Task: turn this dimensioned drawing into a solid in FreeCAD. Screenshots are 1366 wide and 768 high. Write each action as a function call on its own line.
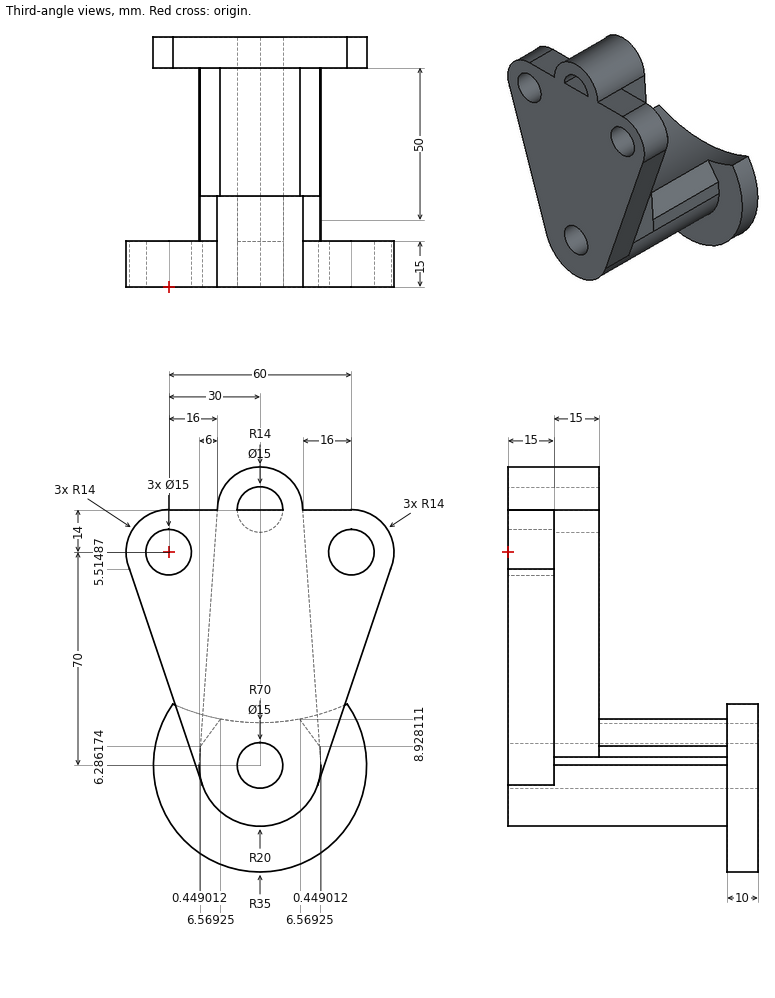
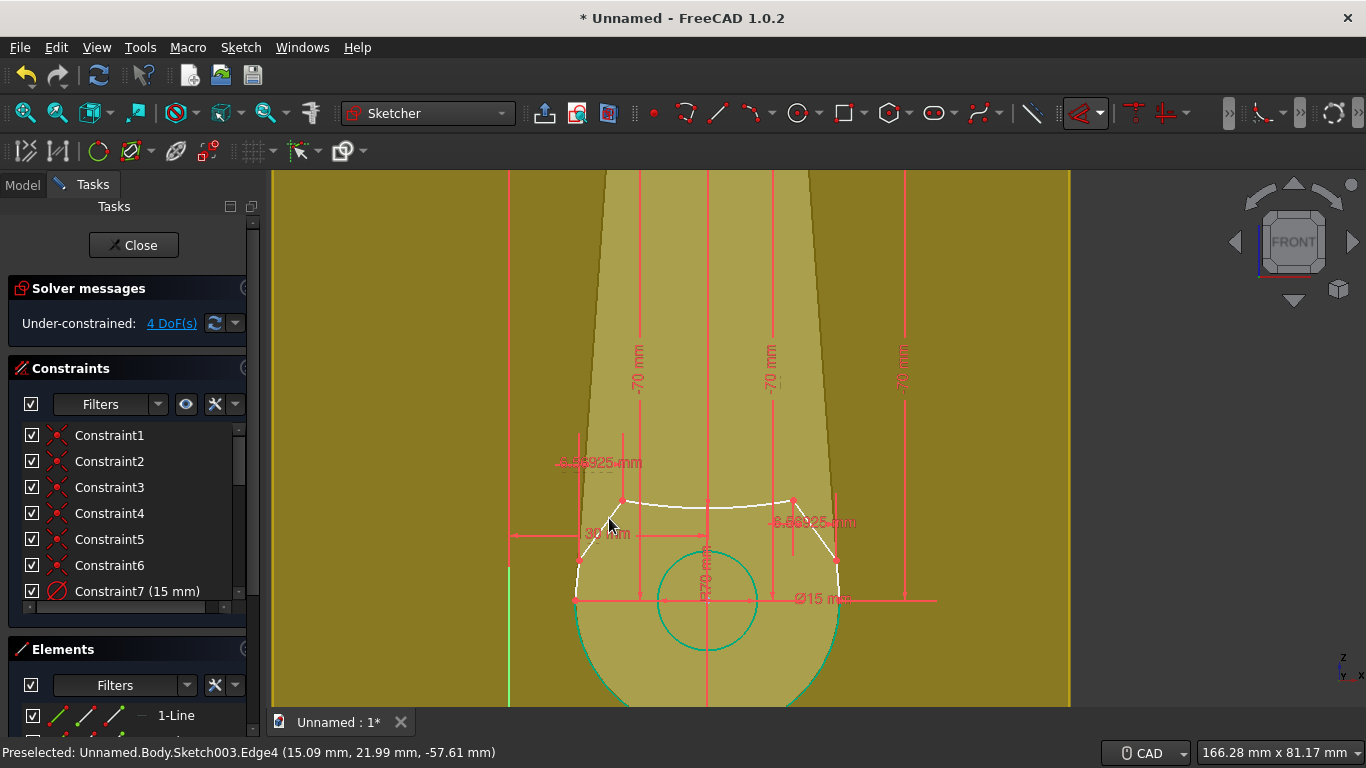
click(823, 542)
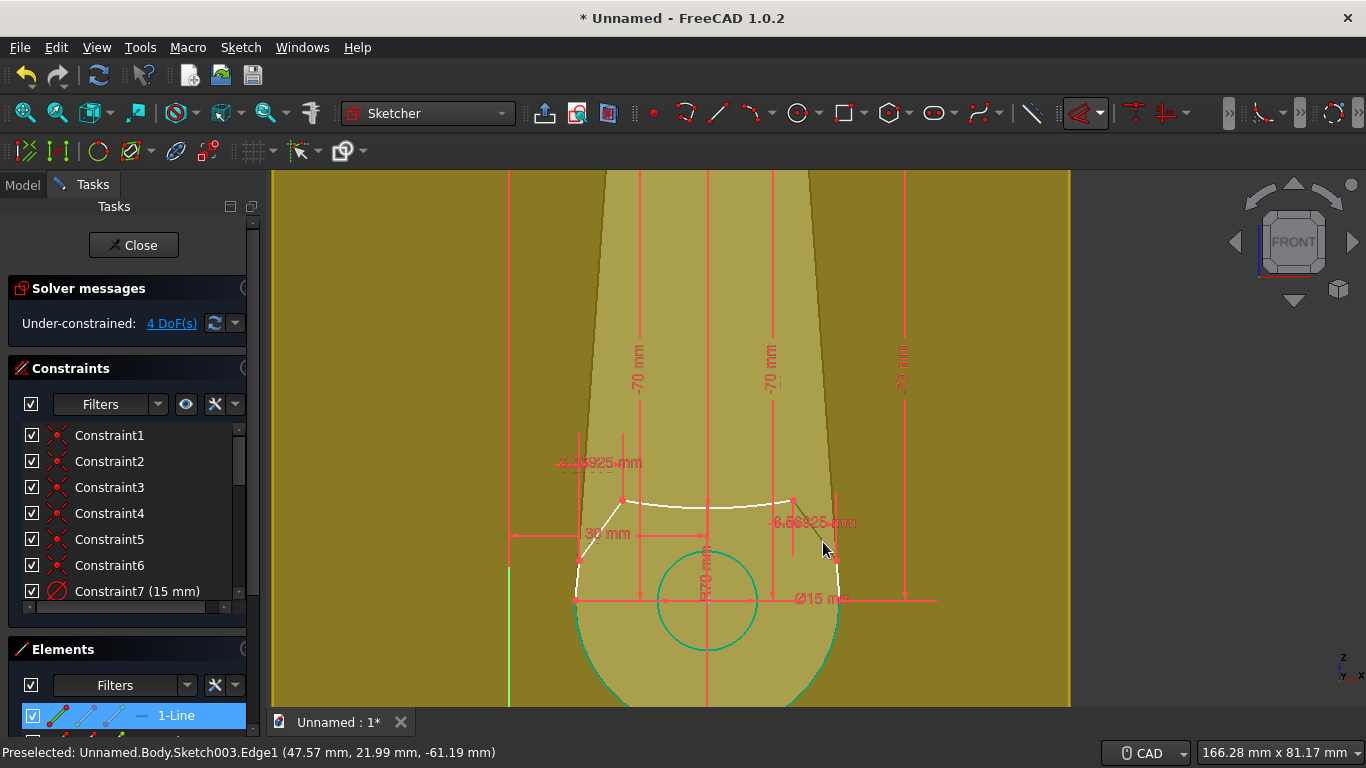
click(1102, 114)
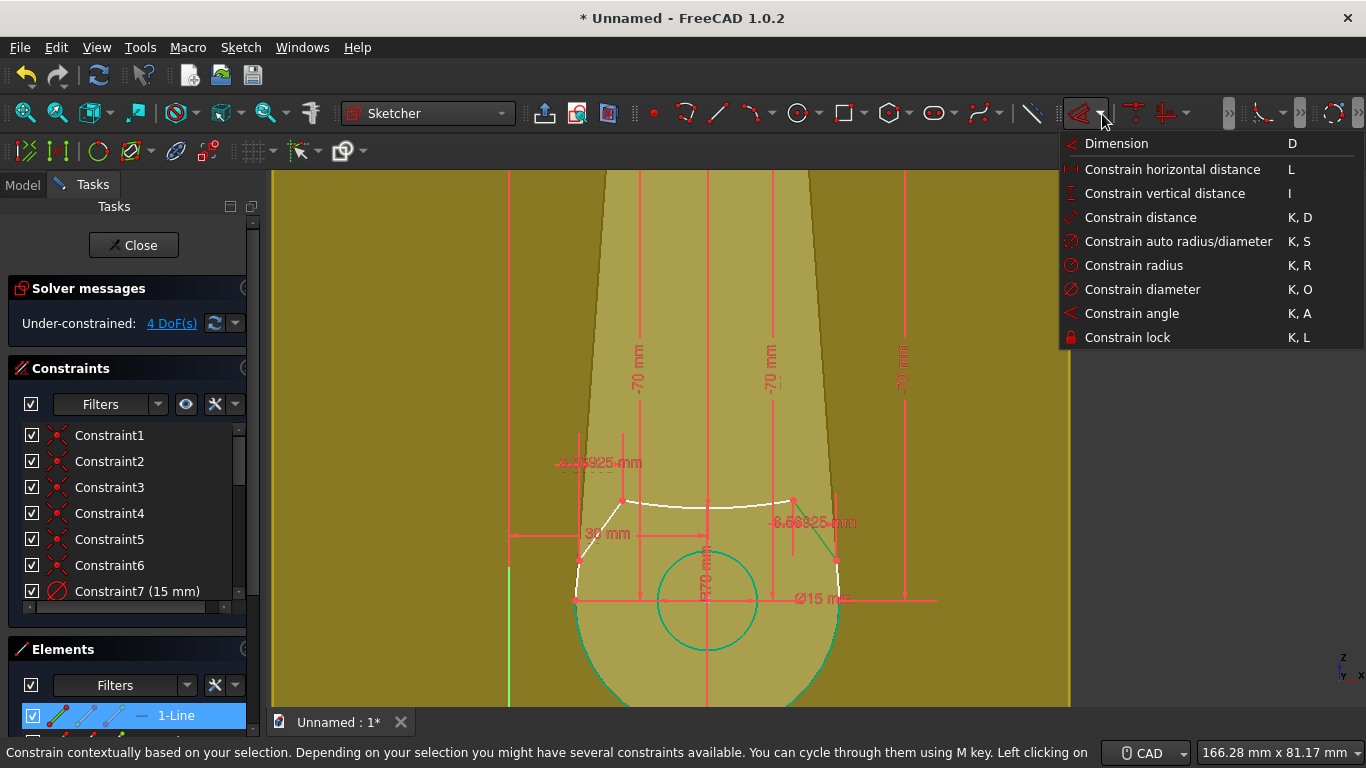
click(1212, 193)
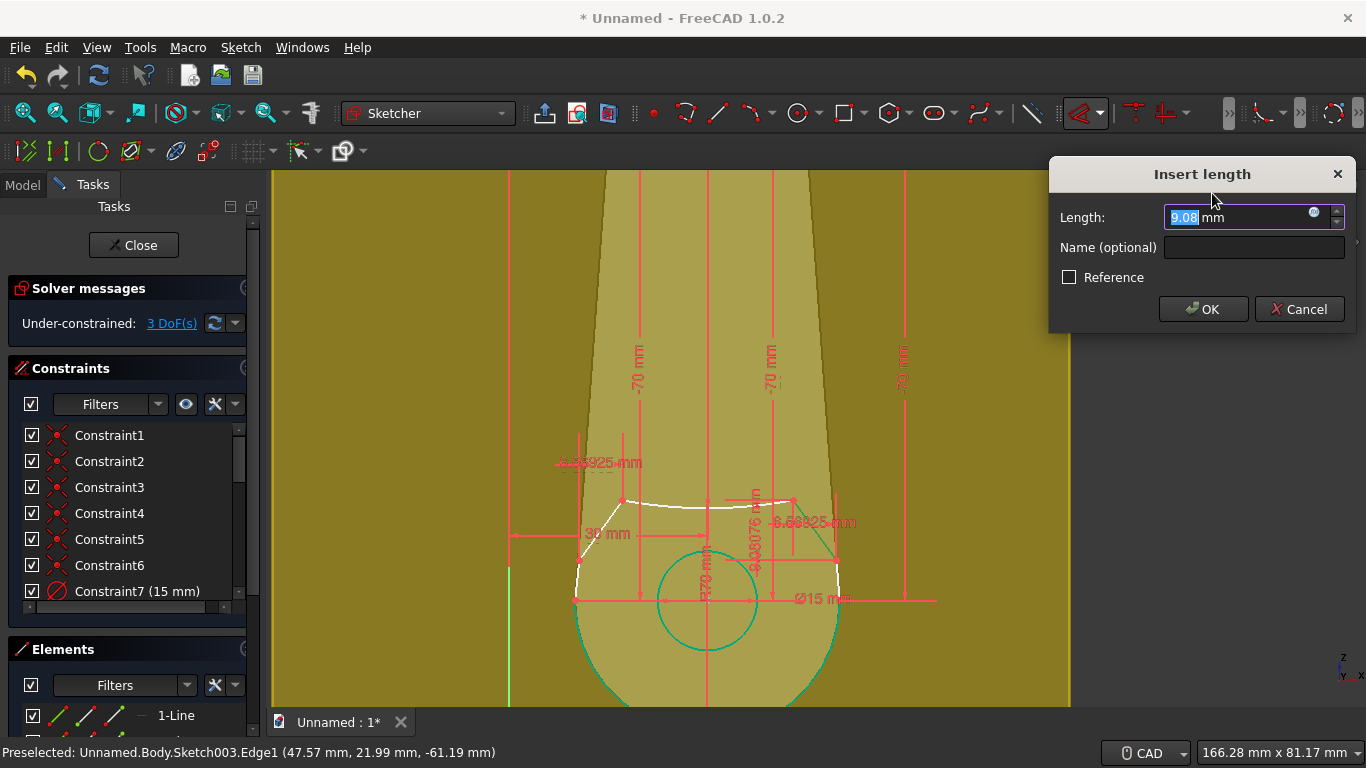
text(8.928111)
key(Return)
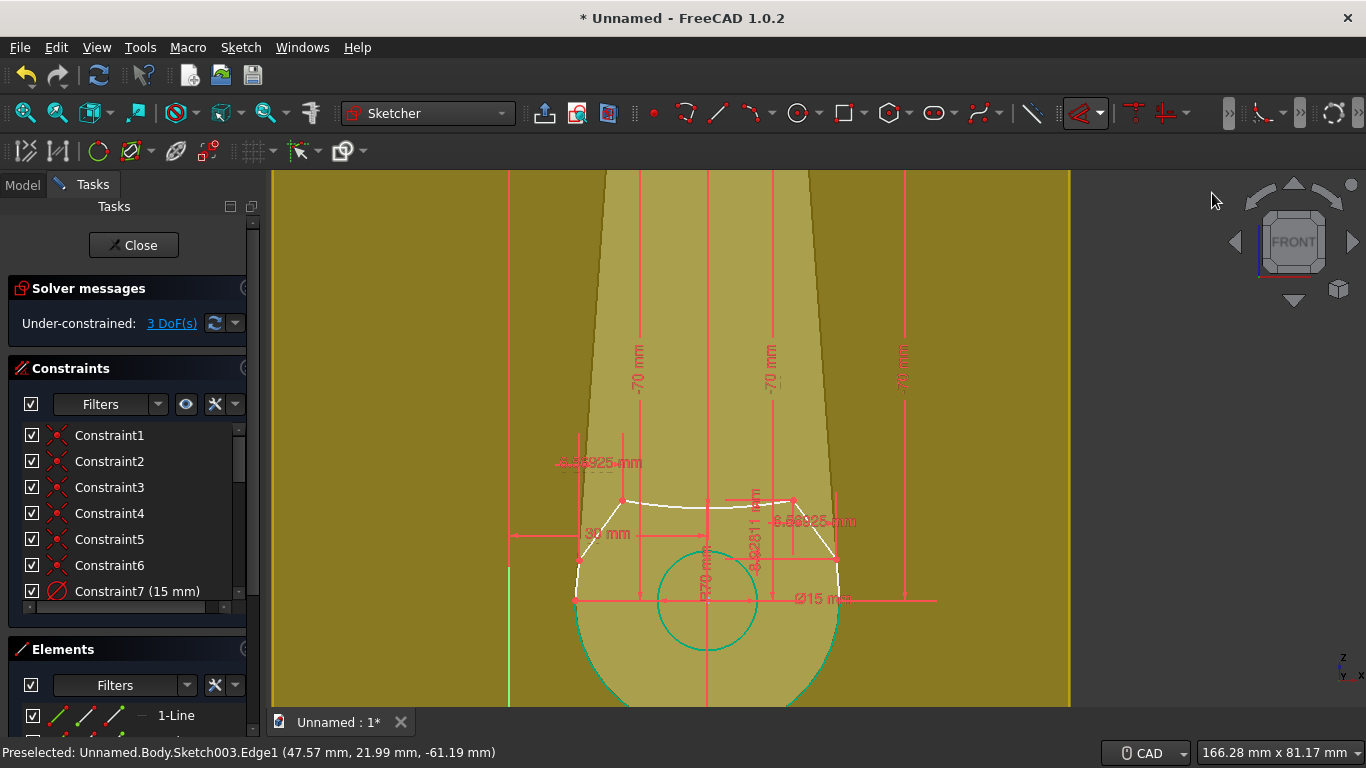
scroll(837, 572, up, 13)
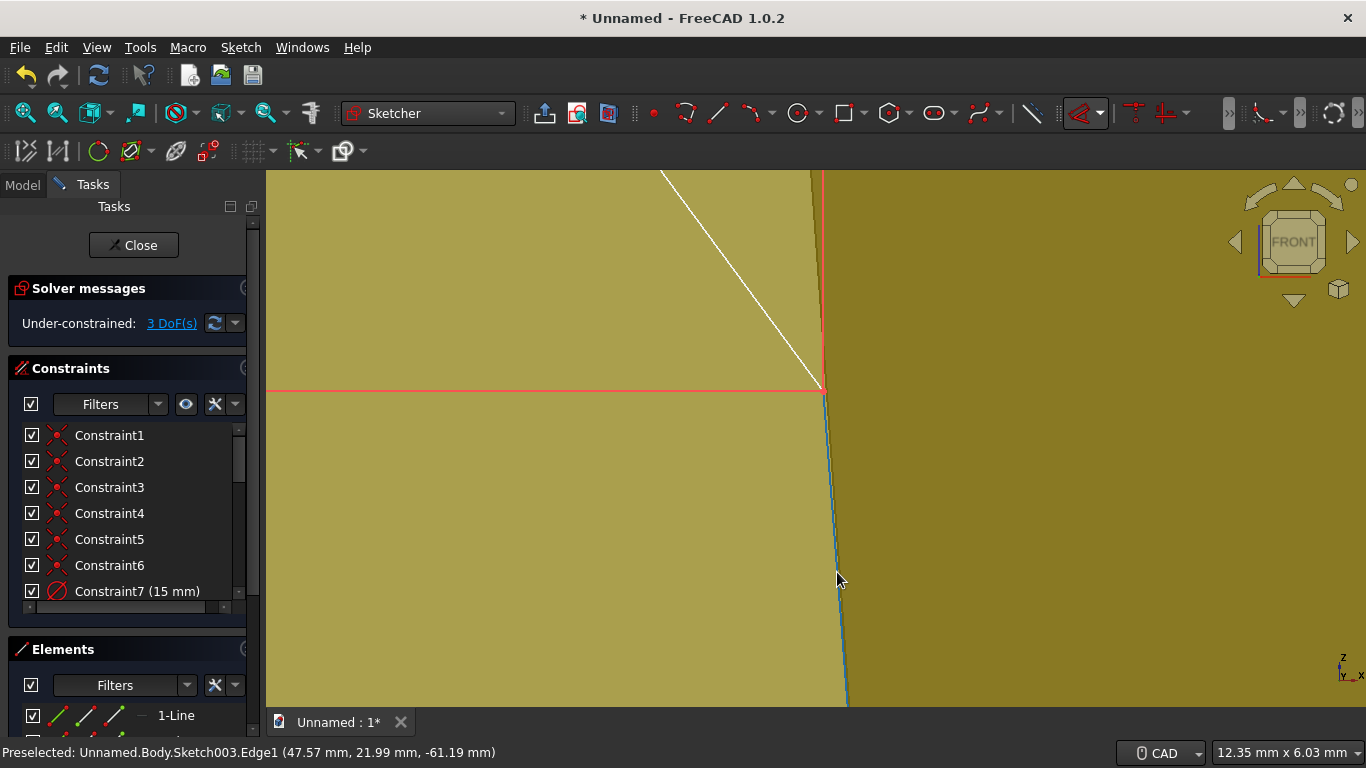
click(836, 559)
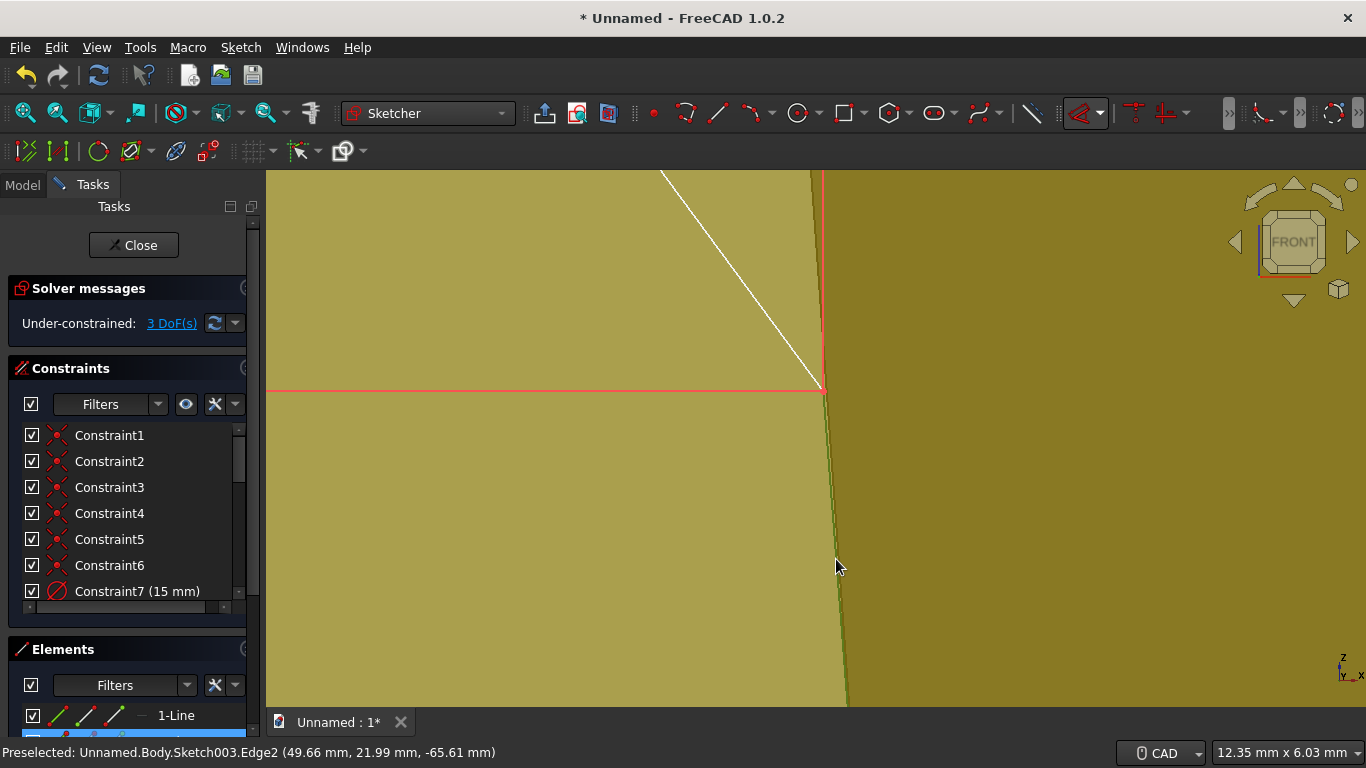
key(l)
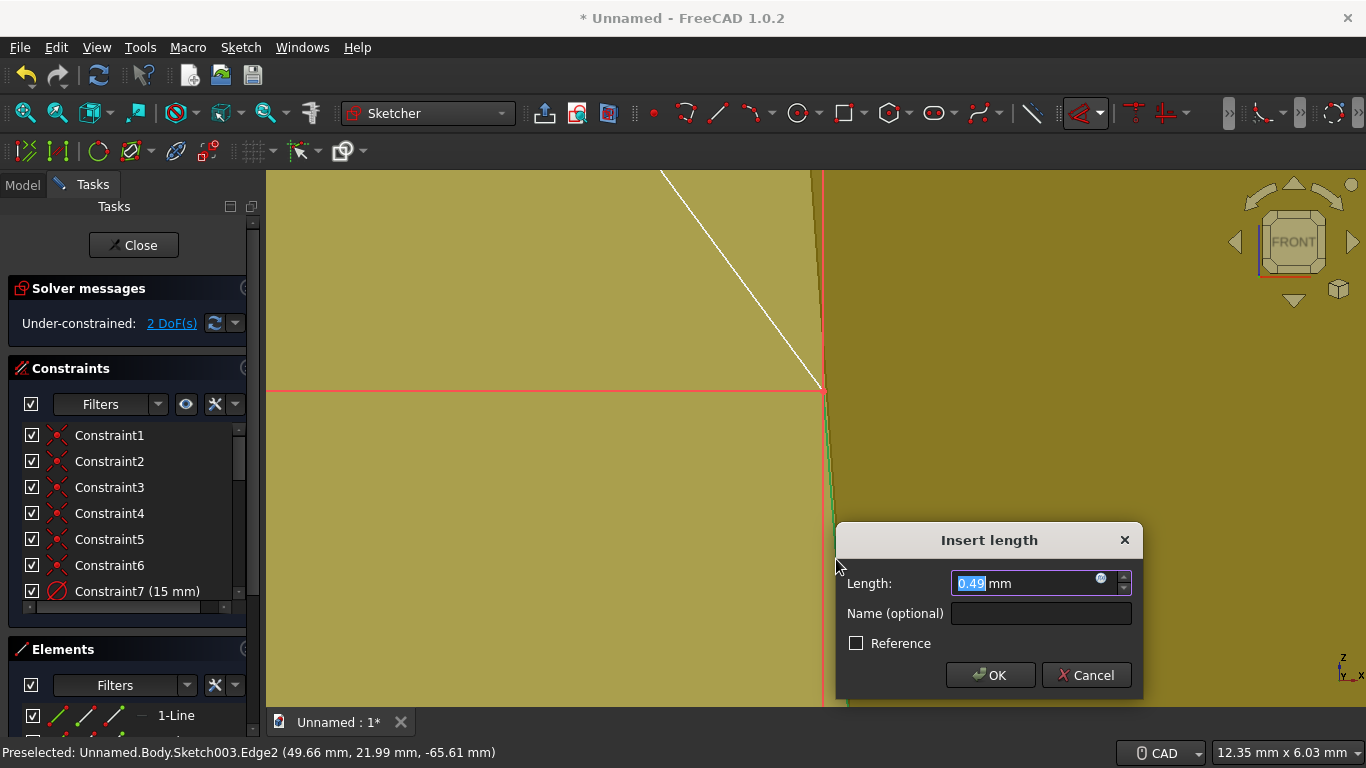
text(0.449012)
key(Return)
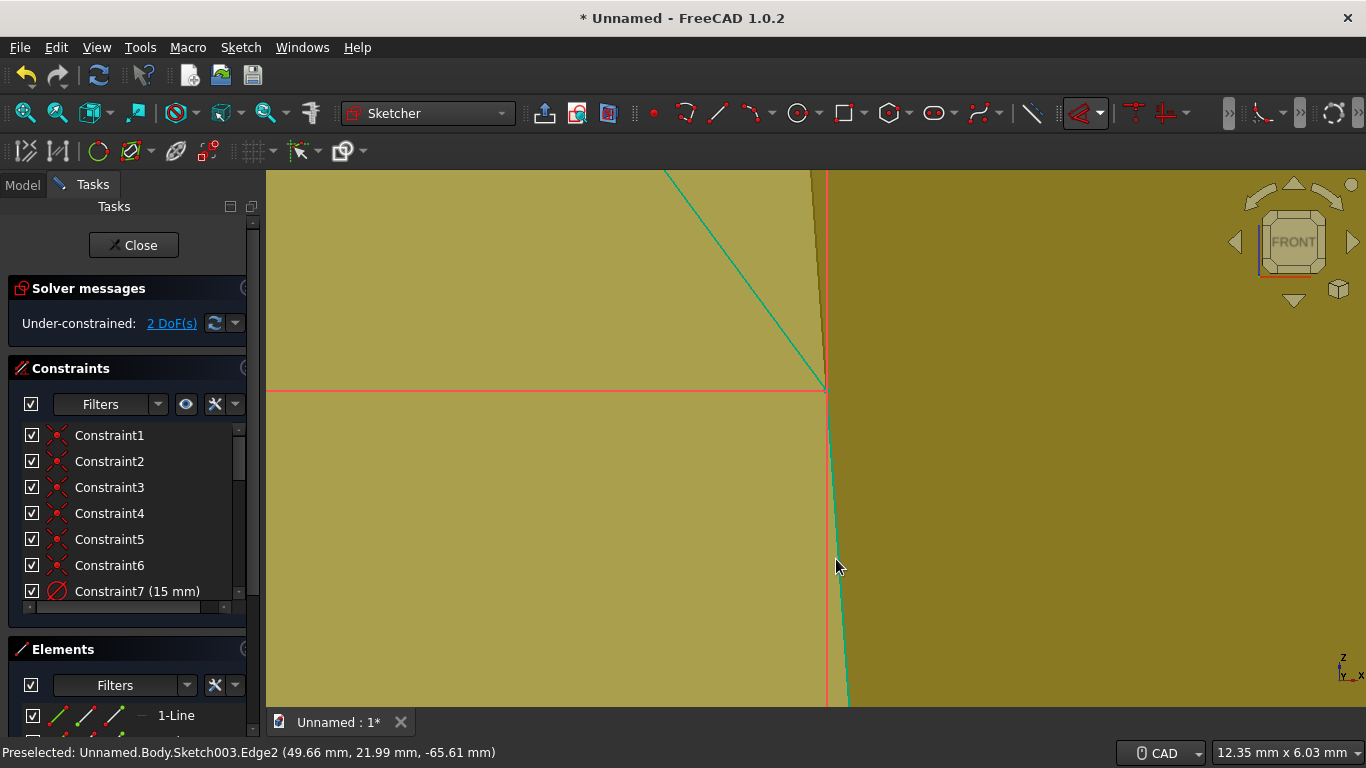
scroll(858, 528, down, 15)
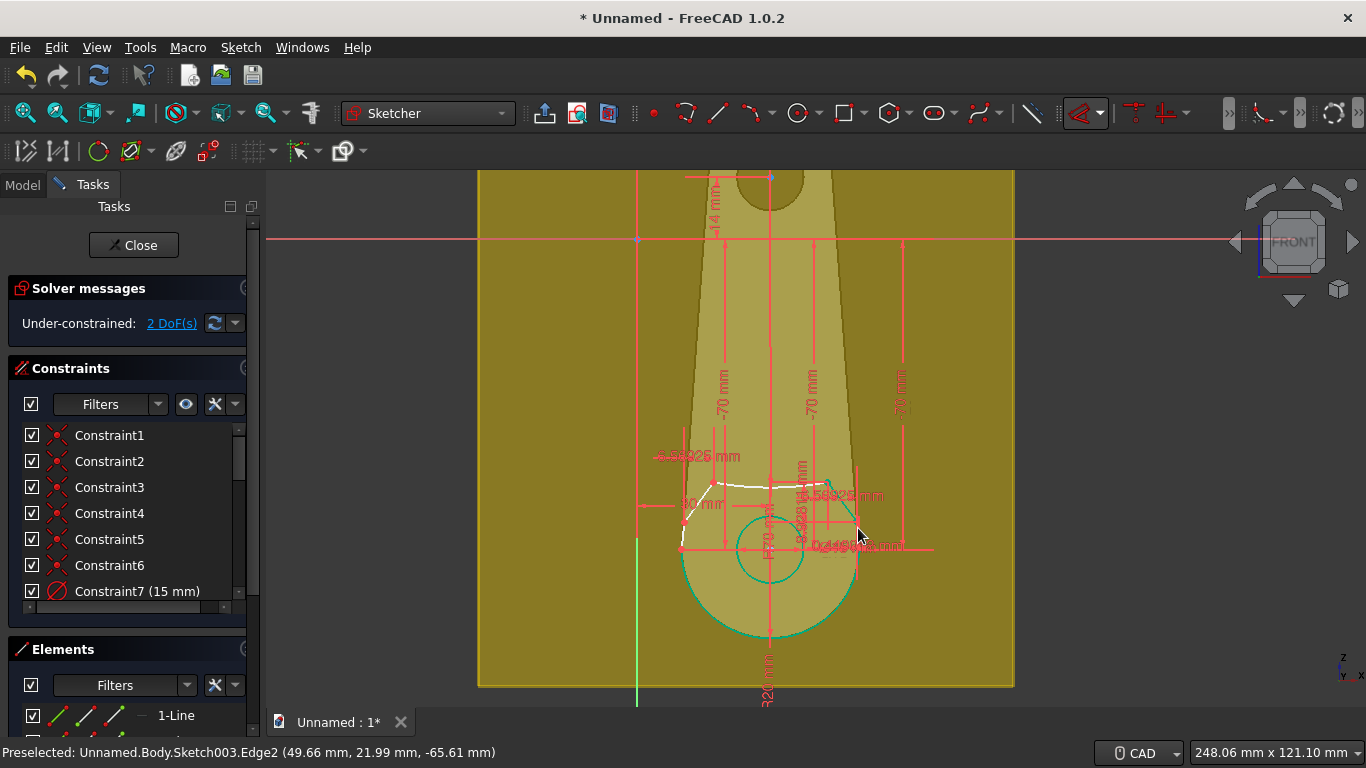
scroll(682, 542, up, 15)